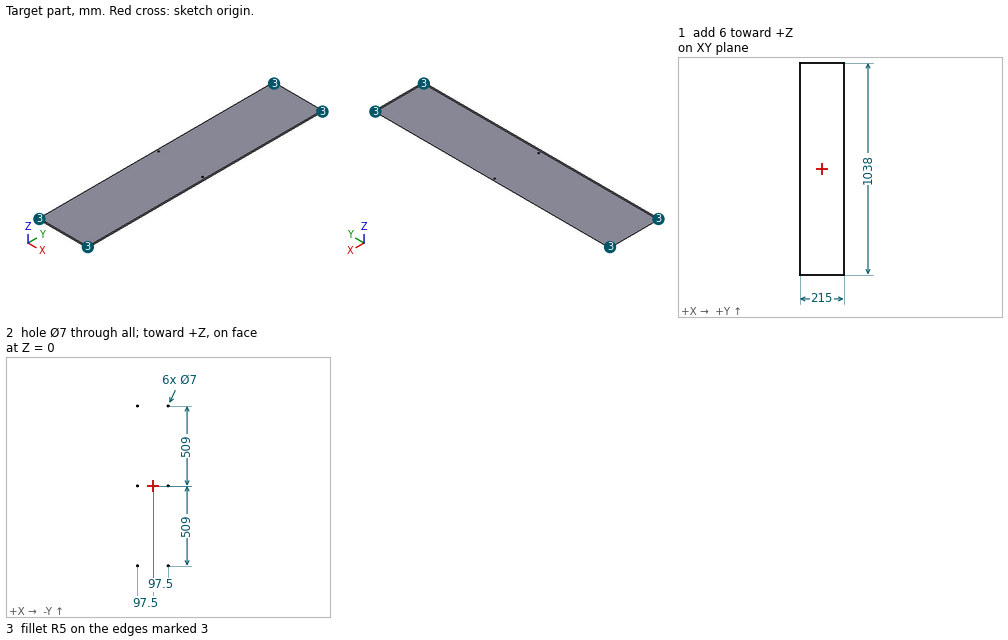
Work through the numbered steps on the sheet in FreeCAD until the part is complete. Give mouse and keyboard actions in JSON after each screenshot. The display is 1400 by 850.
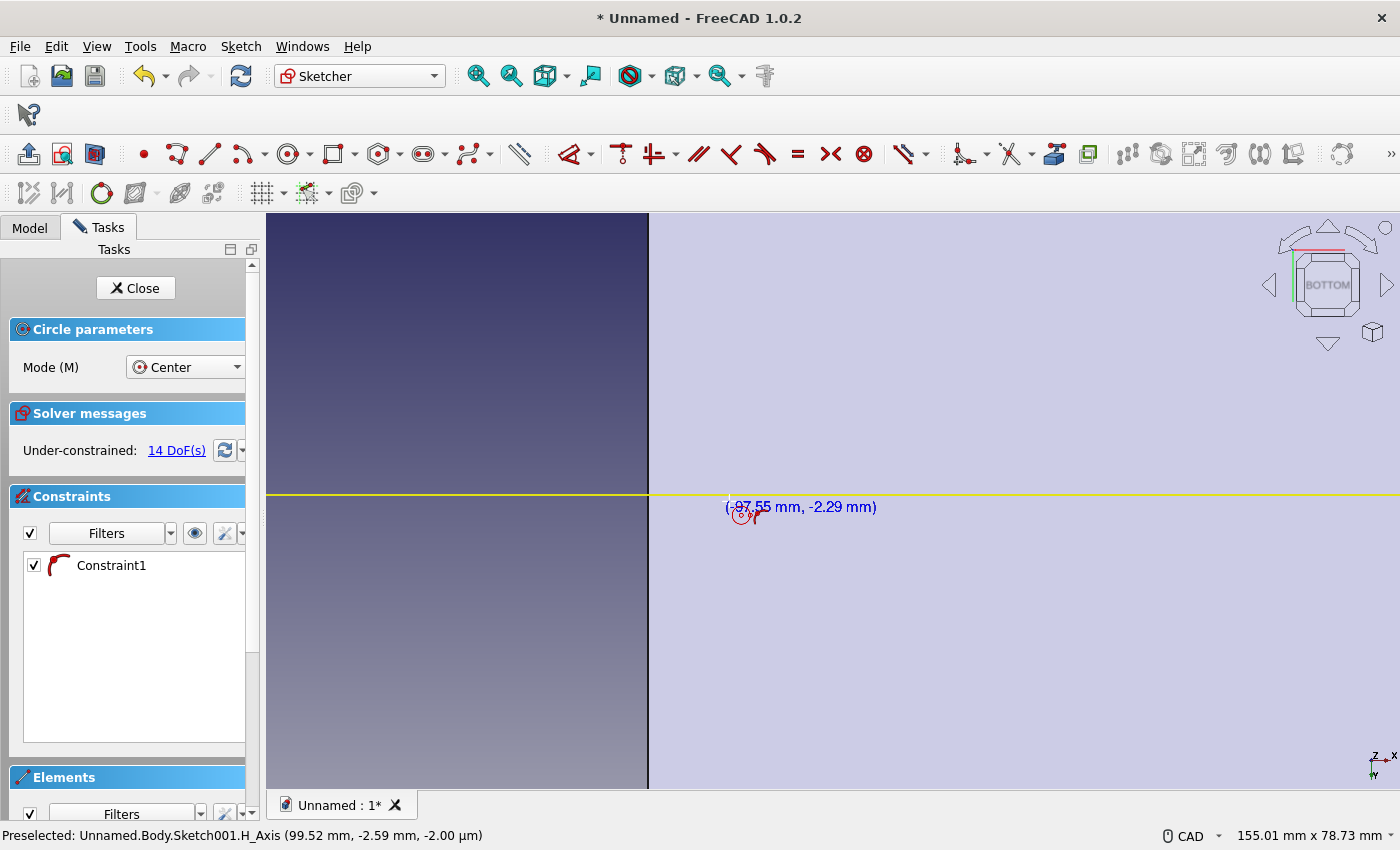
{"action": "scroll", "coordinate": [729, 501], "scroll_direction": "down", "scroll_amount": 15}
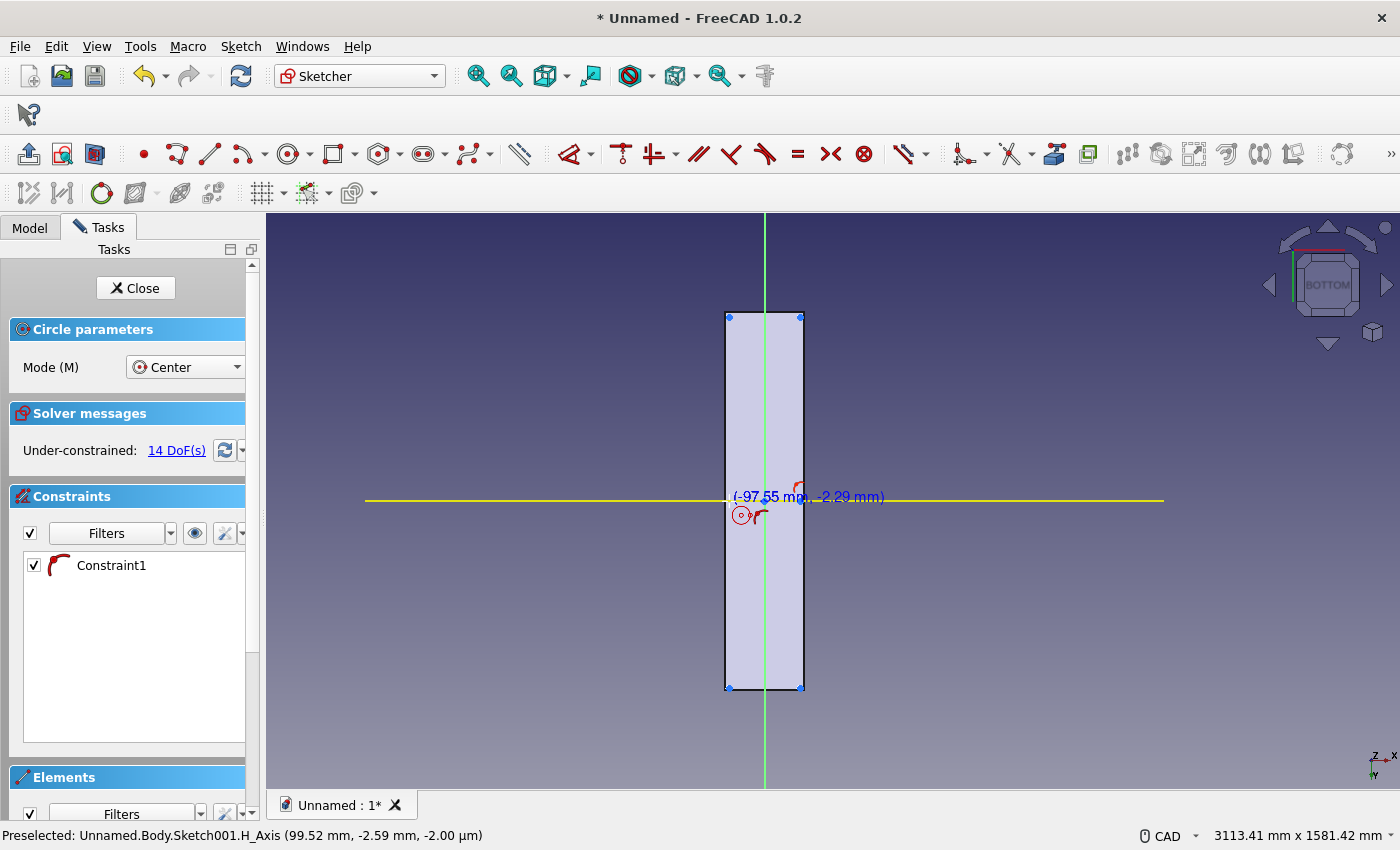
{"action": "left_click", "coordinate": [729, 501]}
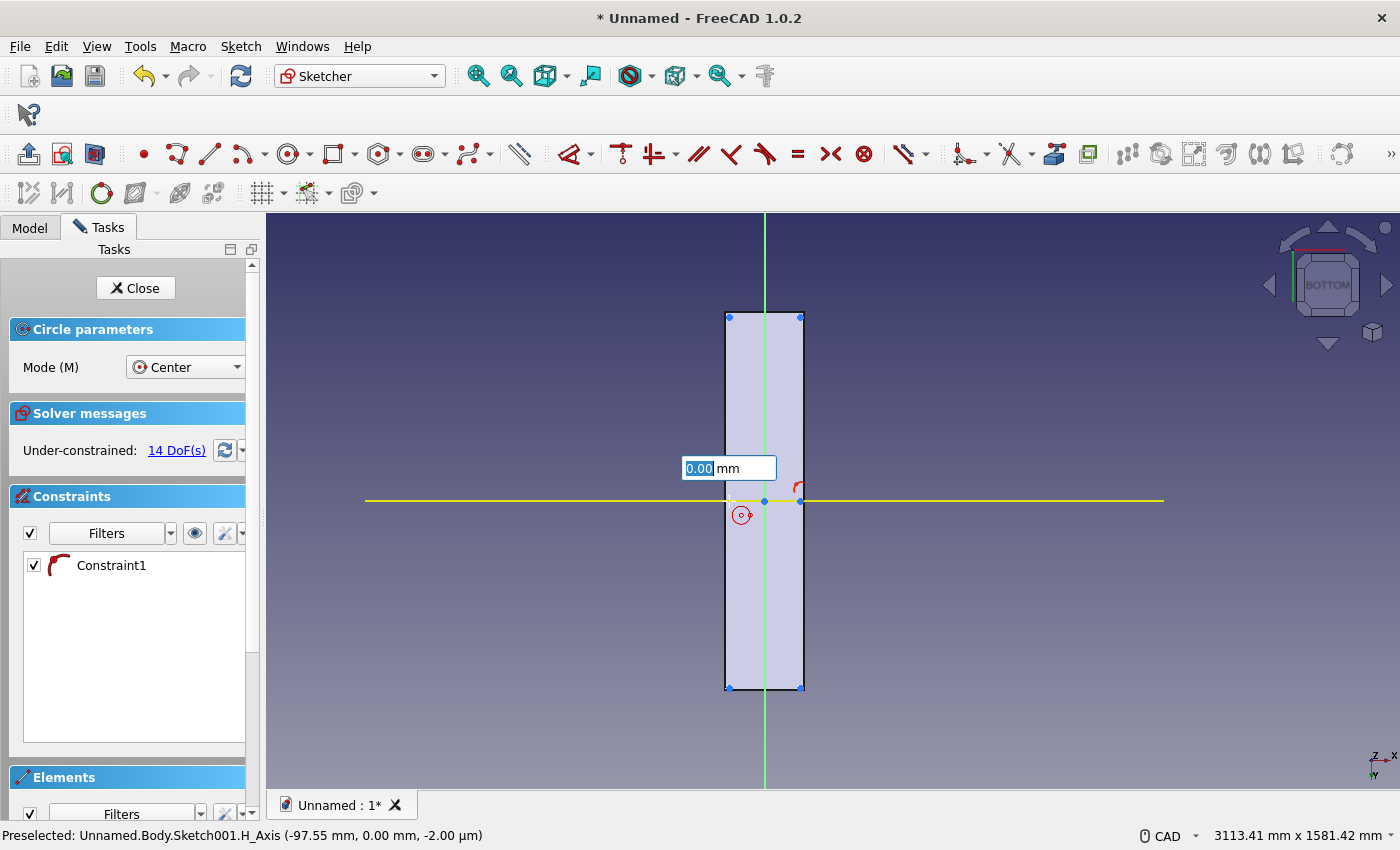
{"action": "scroll", "coordinate": [729, 500], "scroll_direction": "up", "scroll_amount": 13}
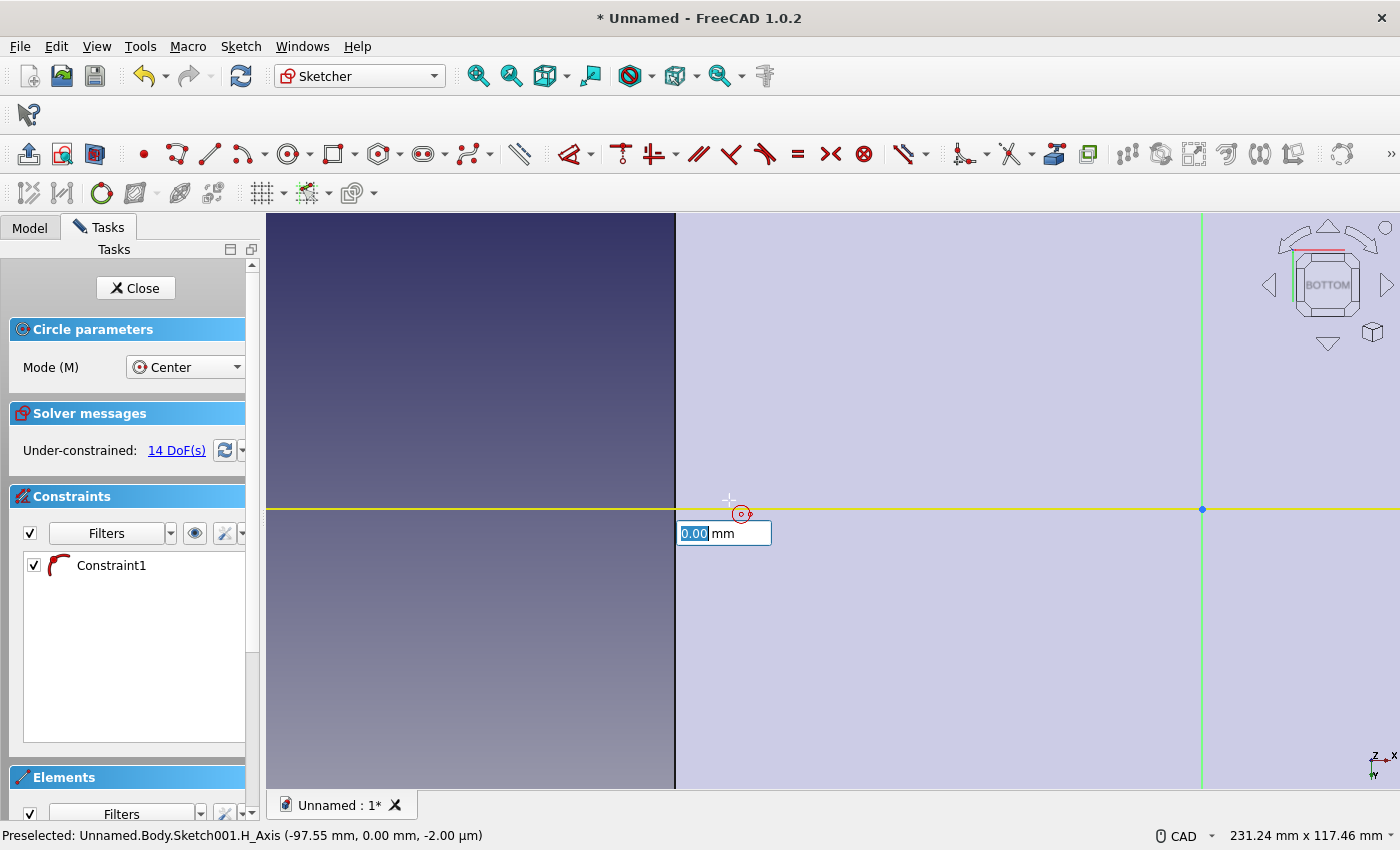
{"action": "left_click", "coordinate": [730, 493]}
{"action": "key", "text": "Escape"}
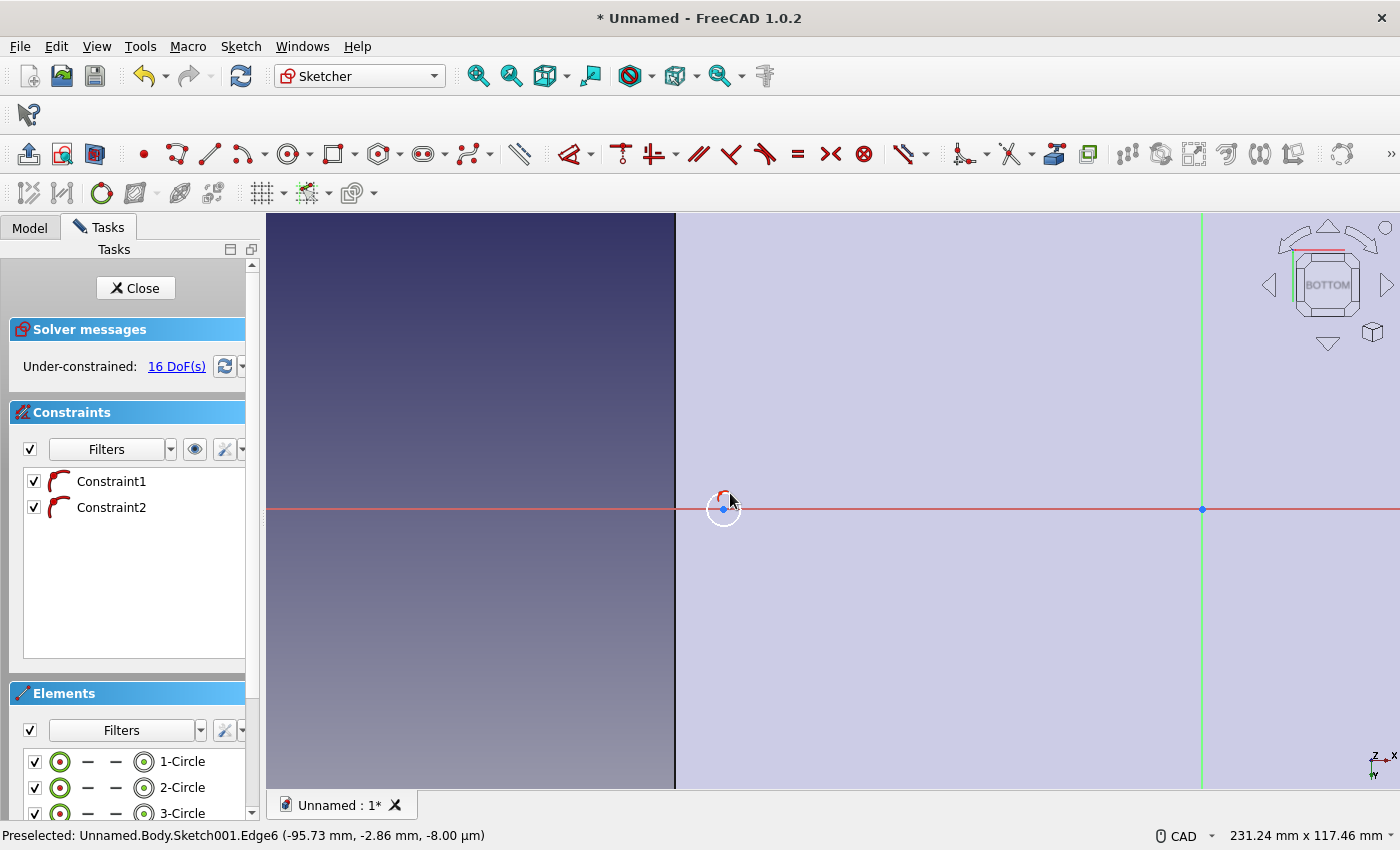
{"action": "scroll", "coordinate": [729, 500], "scroll_direction": "down", "scroll_amount": 13}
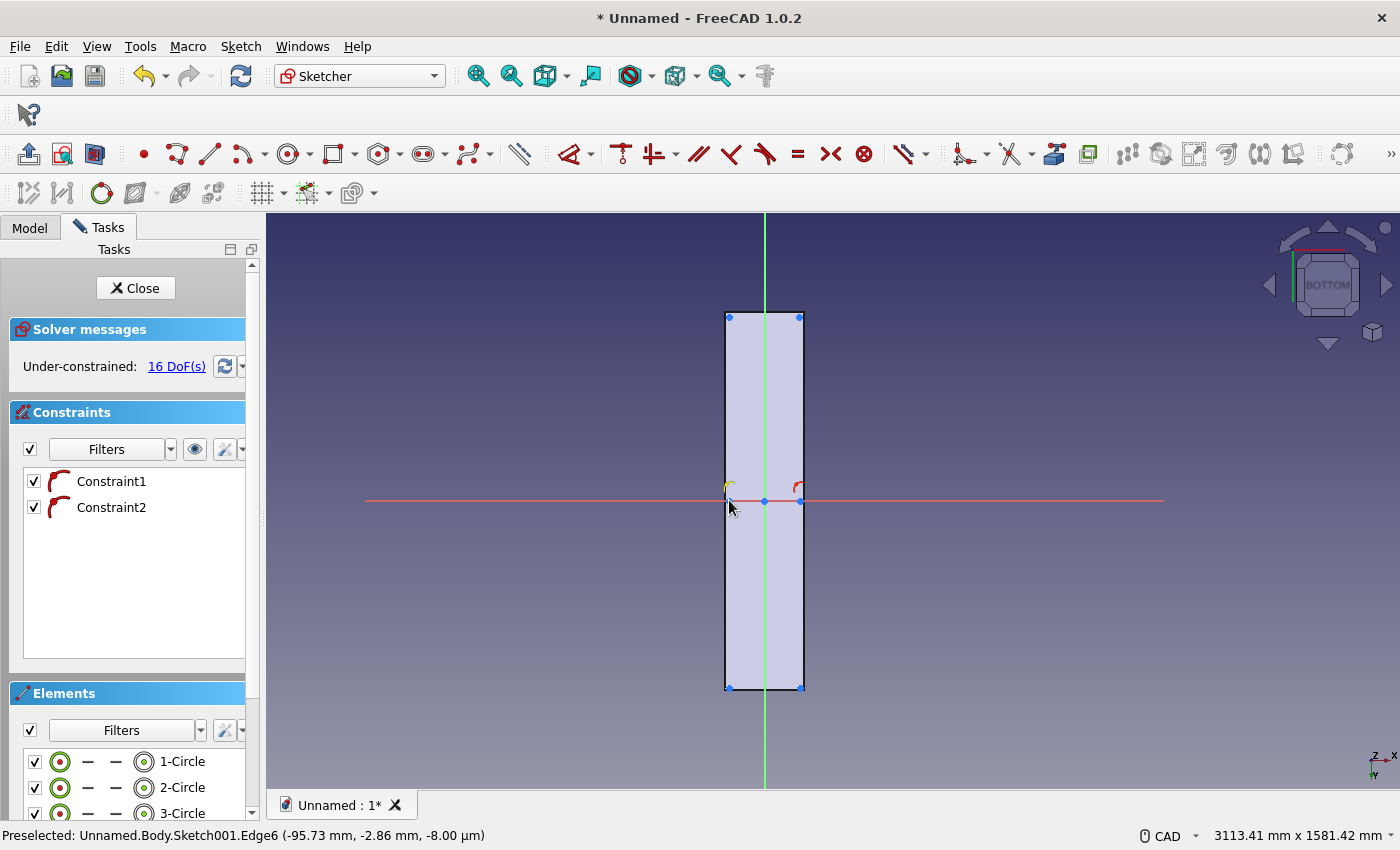
{"action": "scroll", "coordinate": [802, 686], "scroll_direction": "up", "scroll_amount": 9}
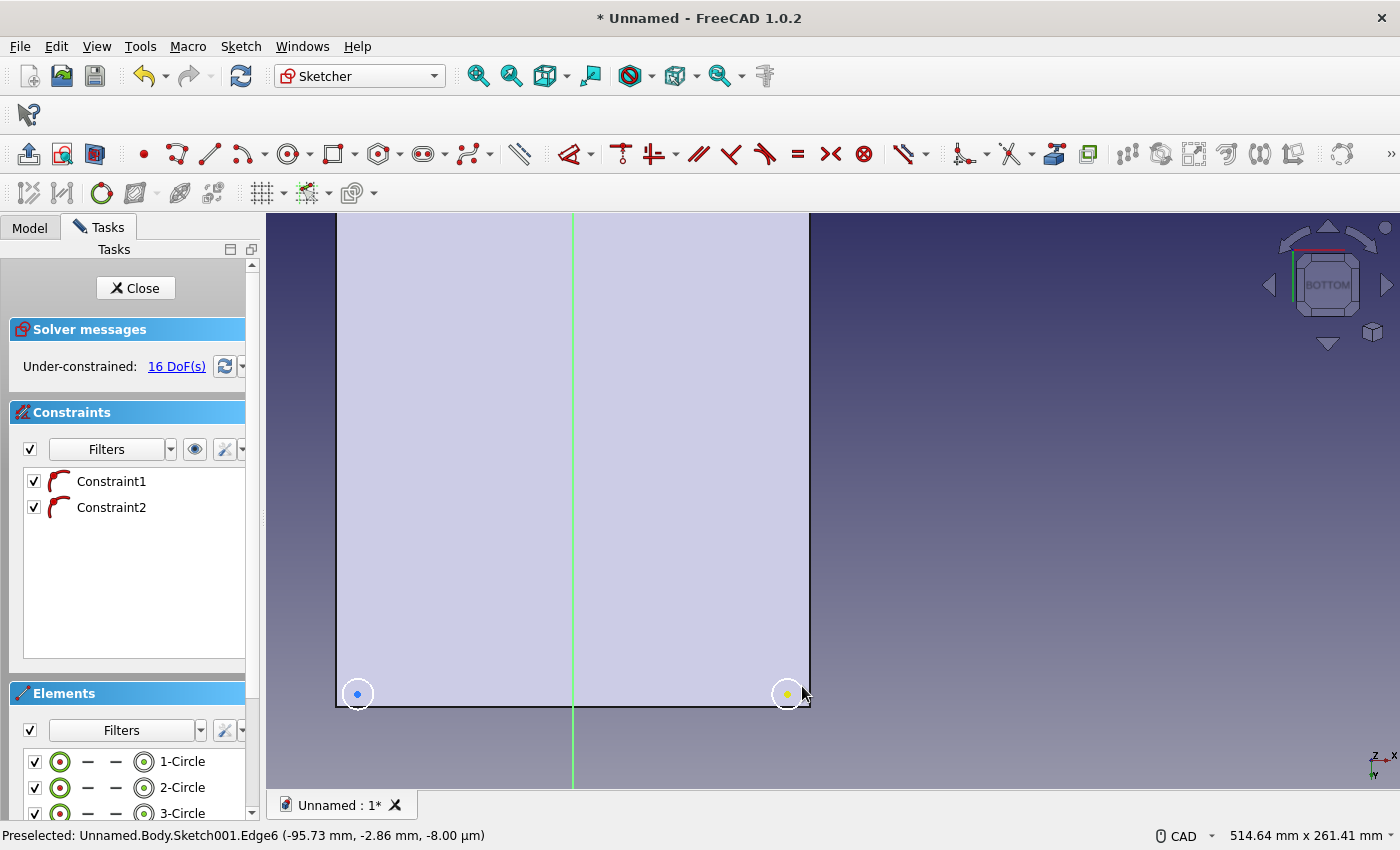
{"action": "left_click", "coordinate": [798, 683]}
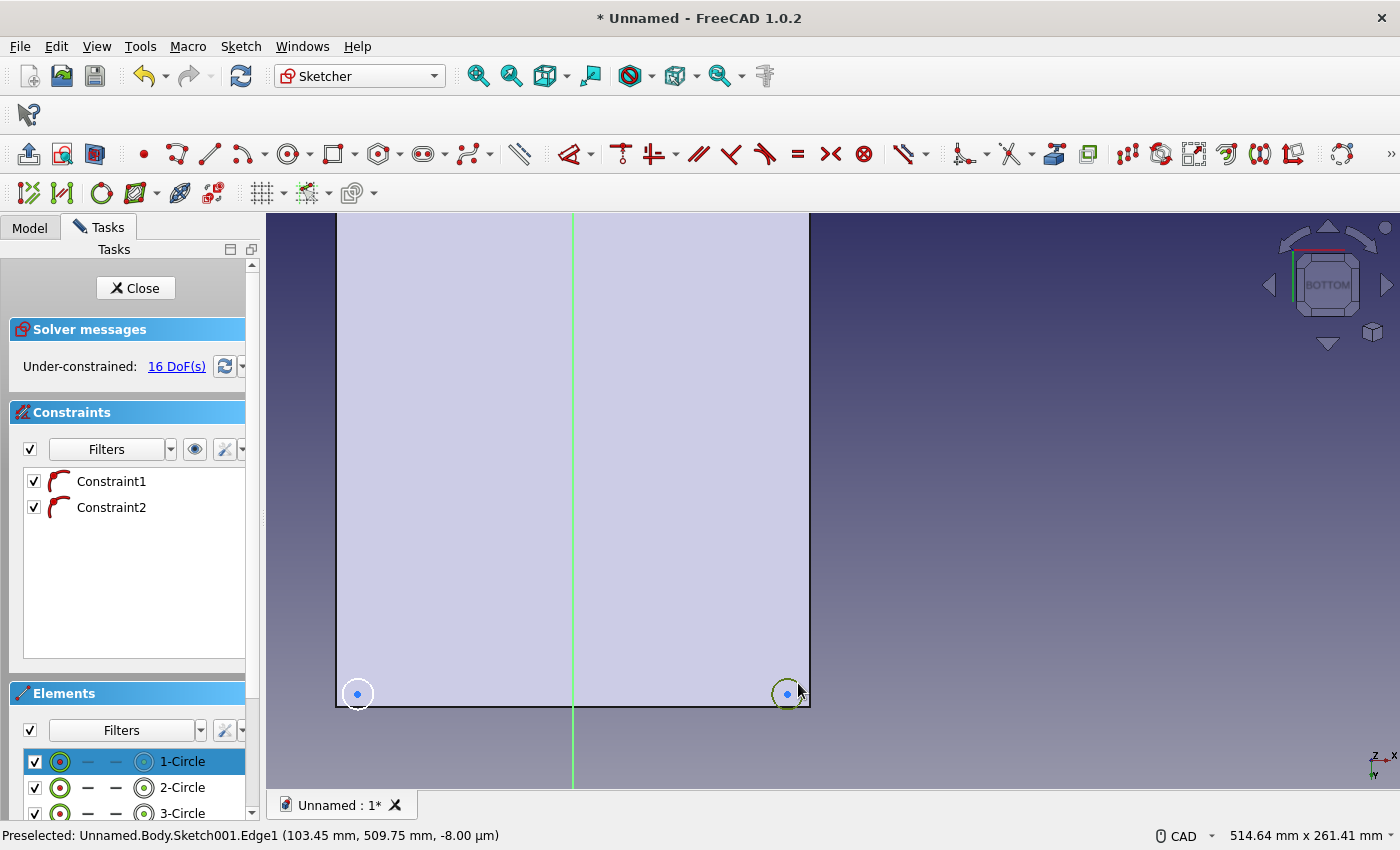
{"action": "scroll", "coordinate": [802, 687], "scroll_direction": "down", "scroll_amount": 9}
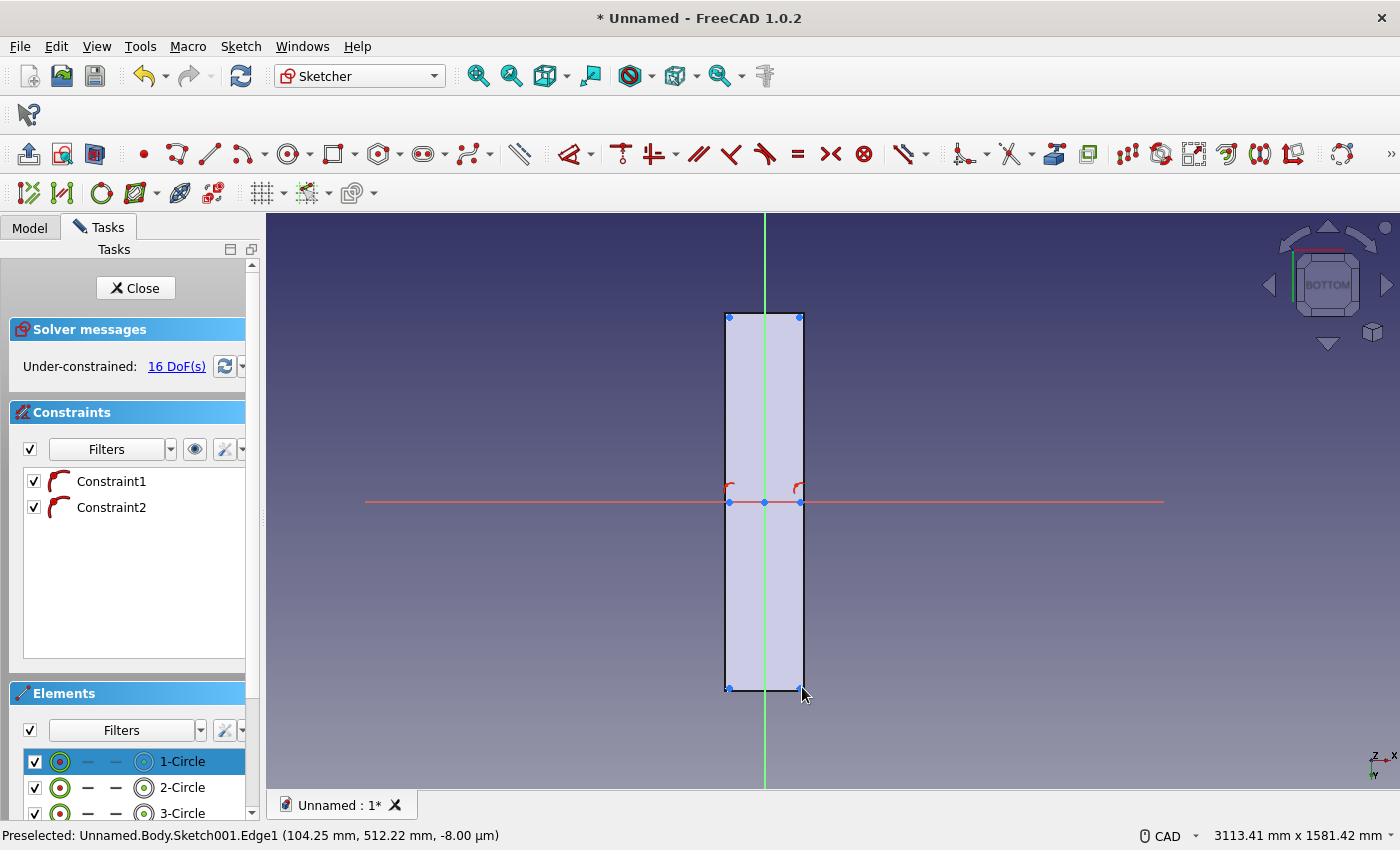
{"action": "scroll", "coordinate": [802, 316], "scroll_direction": "up", "scroll_amount": 10}